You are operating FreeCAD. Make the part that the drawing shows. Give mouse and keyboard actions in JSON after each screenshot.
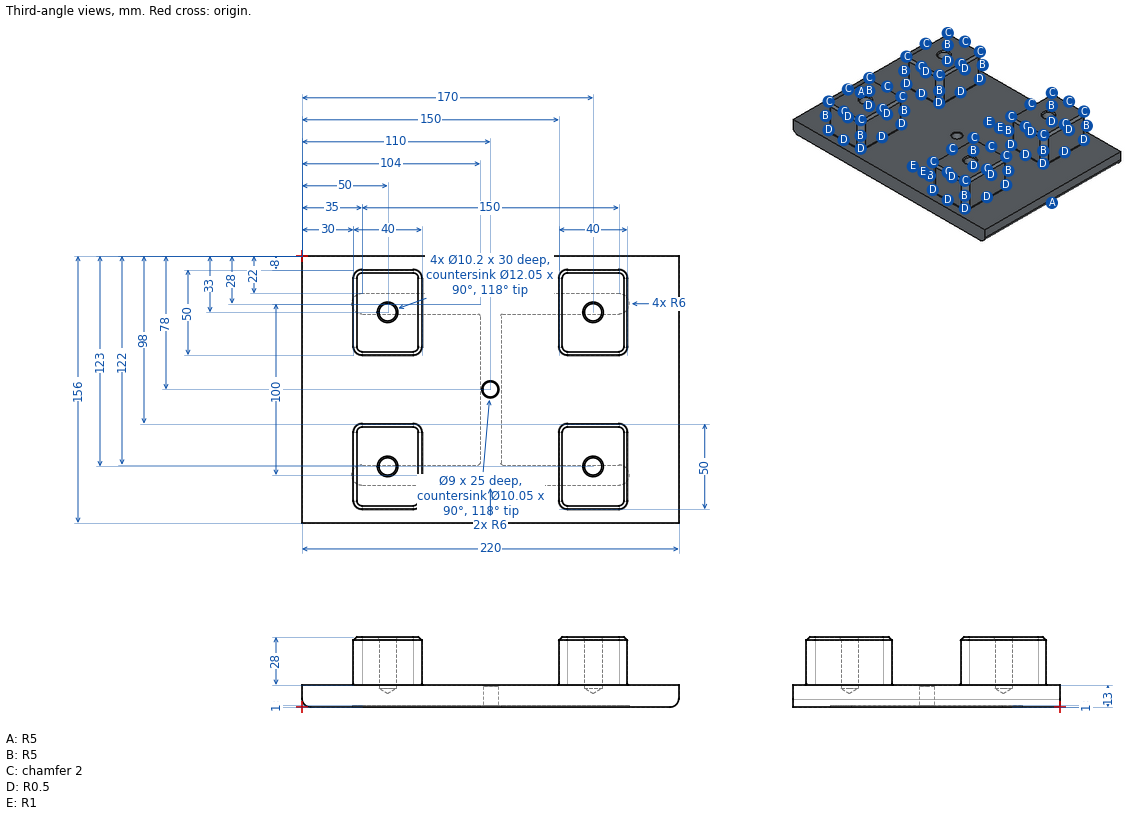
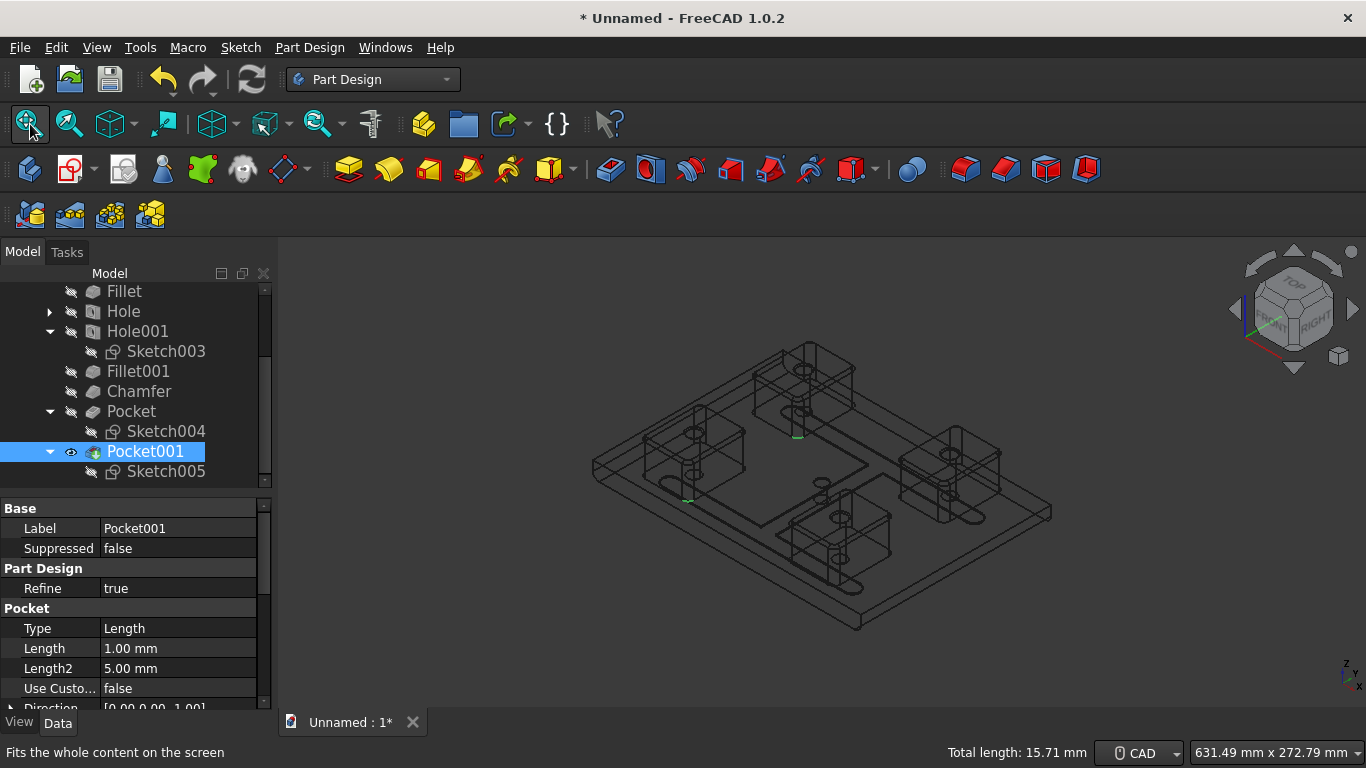
{"action": "left_click", "coordinate": [725, 453], "text": "ctrl"}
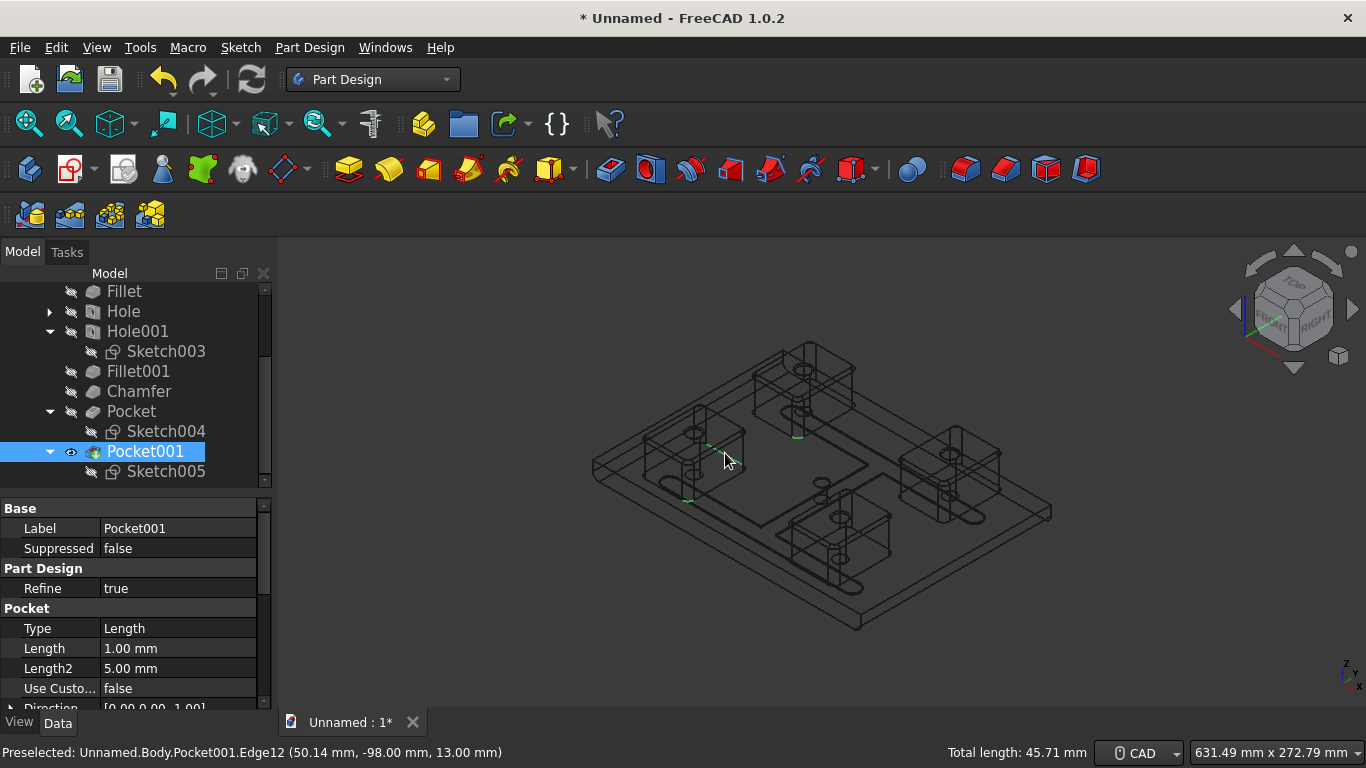
{"action": "left_click", "coordinate": [718, 485], "text": "ctrl"}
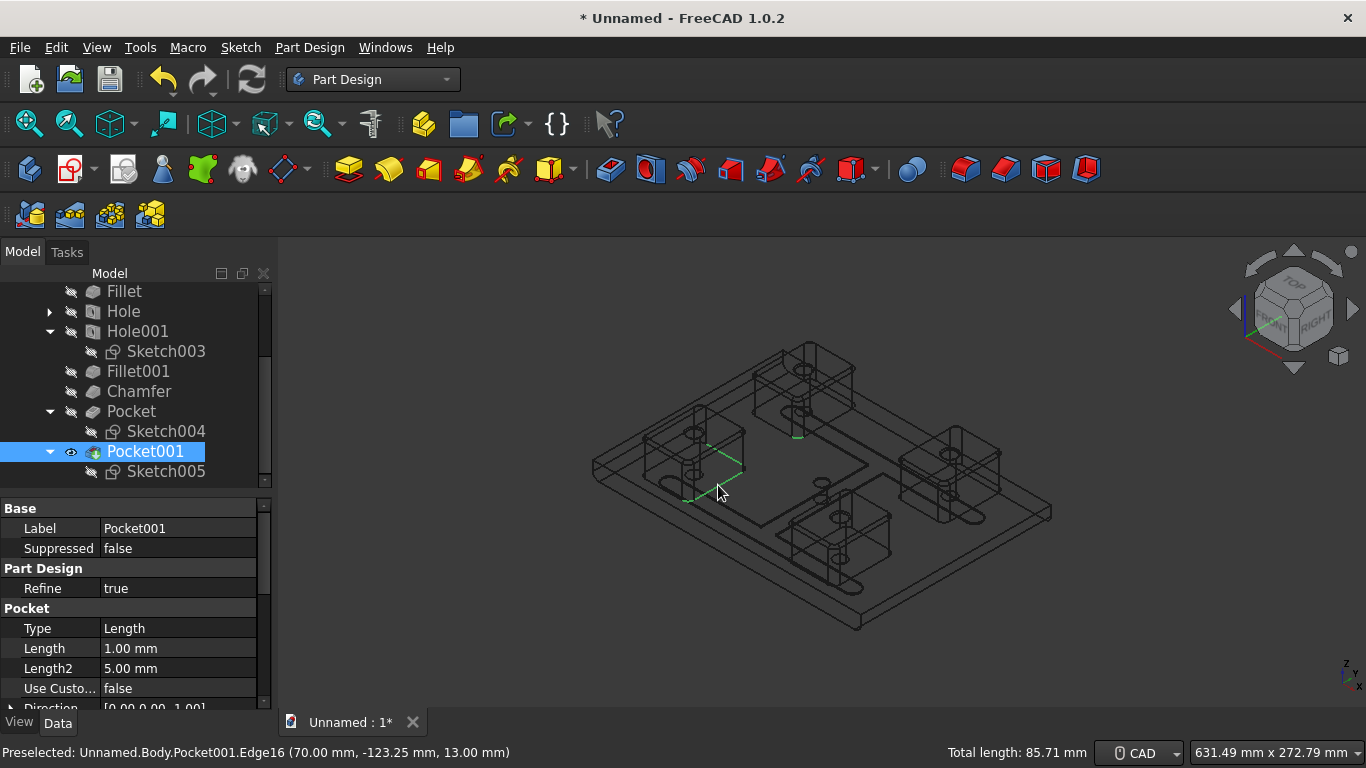
{"action": "left_click", "coordinate": [660, 463], "text": "ctrl"}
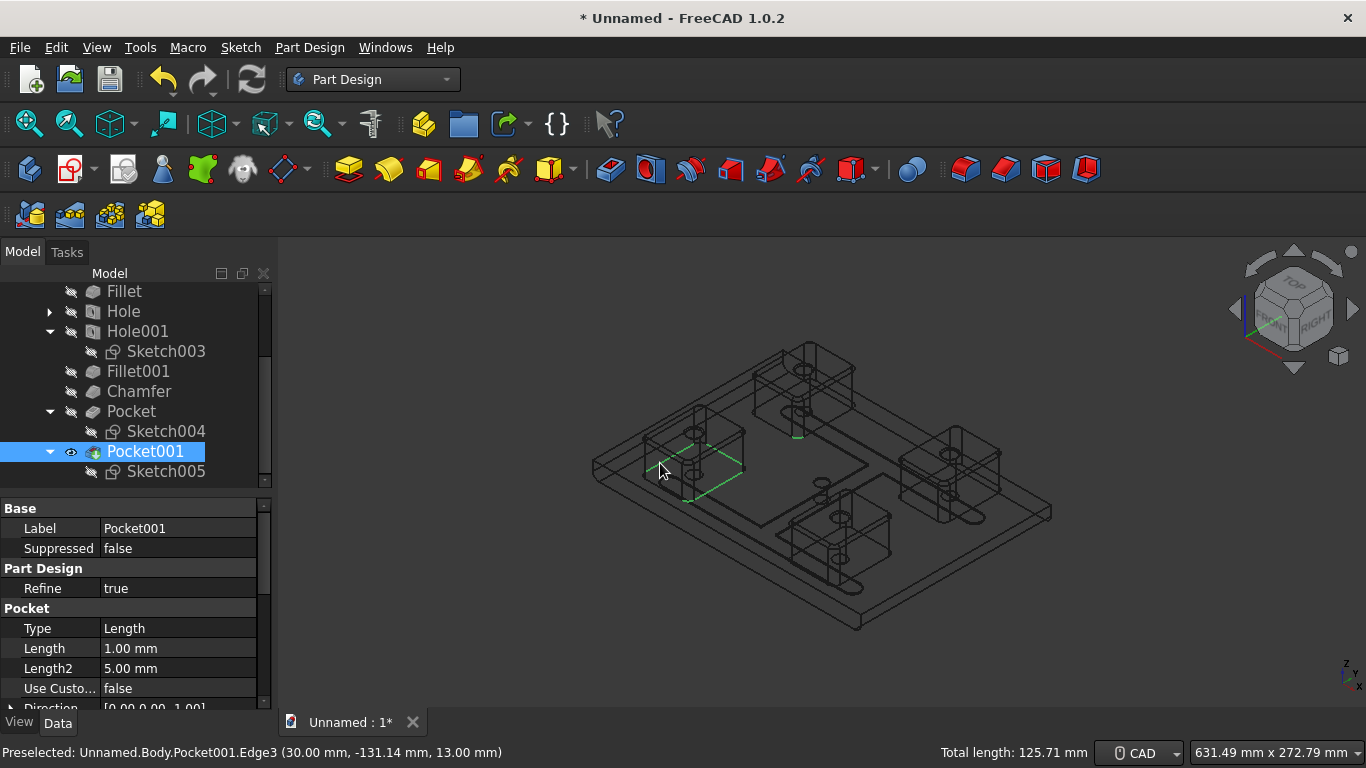
{"action": "left_click", "coordinate": [664, 489], "text": "ctrl"}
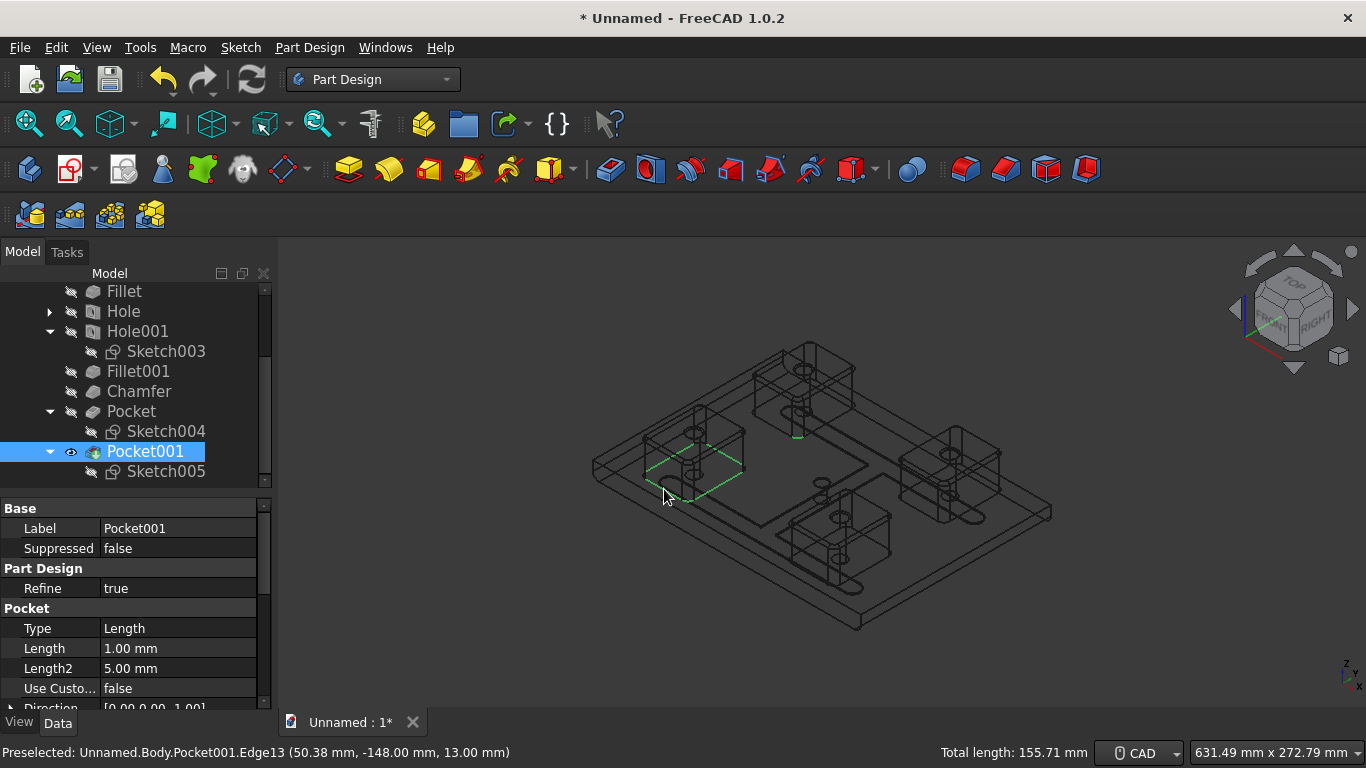
{"action": "left_click", "coordinate": [810, 573], "text": "ctrl"}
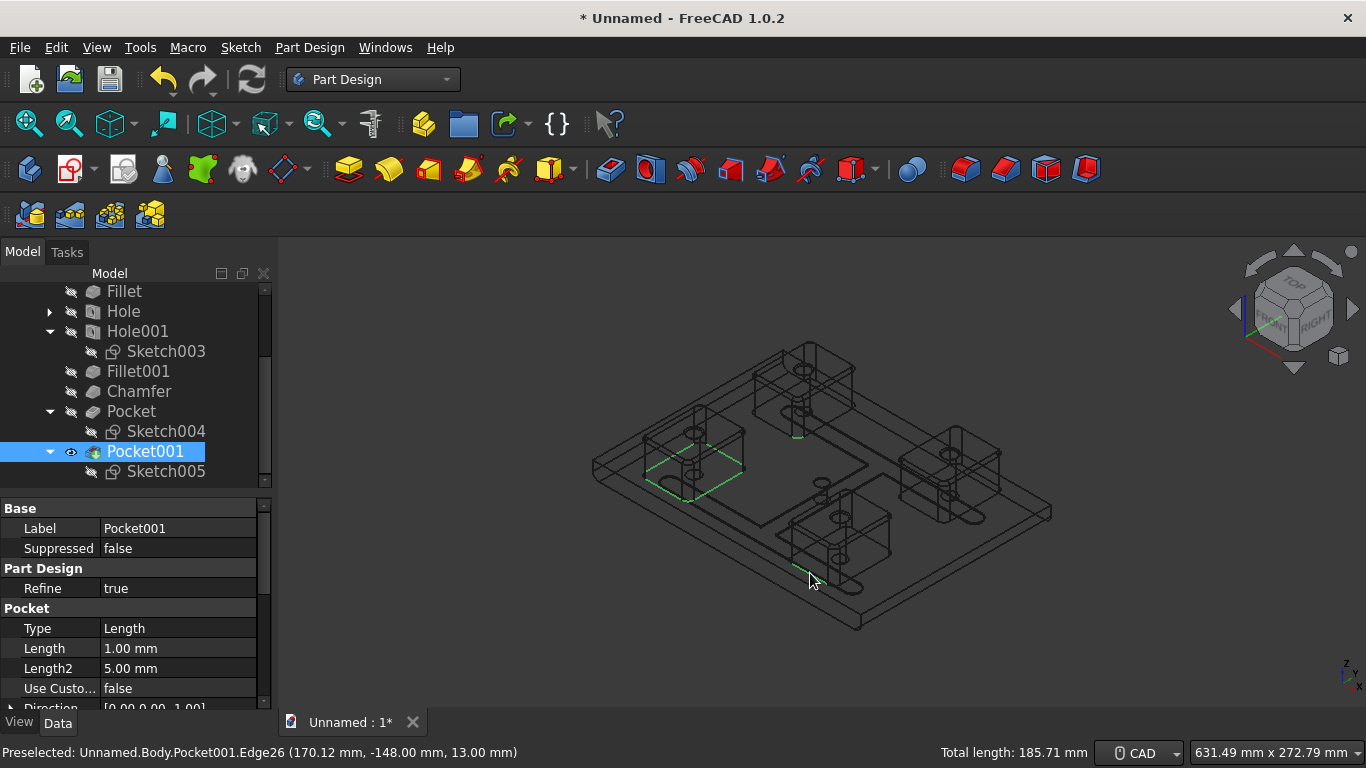
{"action": "left_click", "coordinate": [806, 547], "text": "ctrl"}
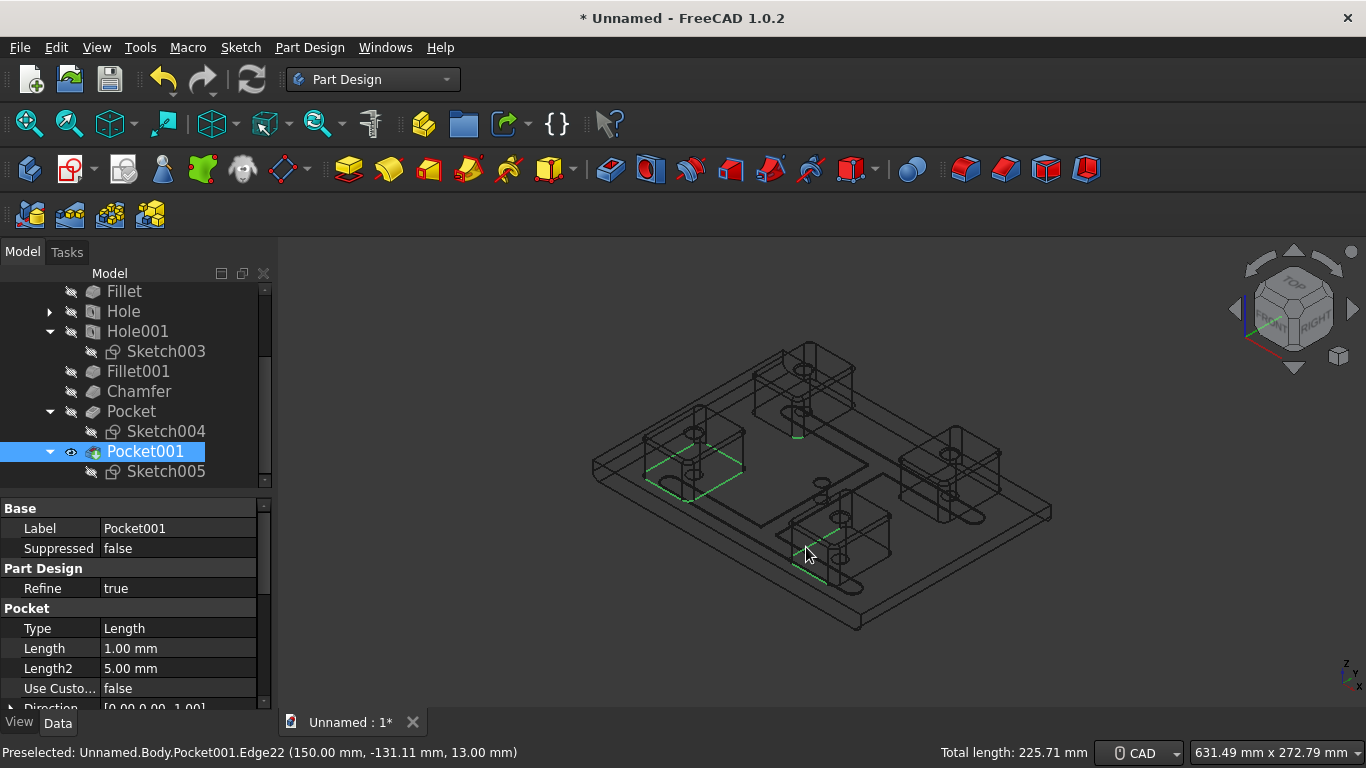
{"action": "left_click", "coordinate": [865, 569], "text": "ctrl"}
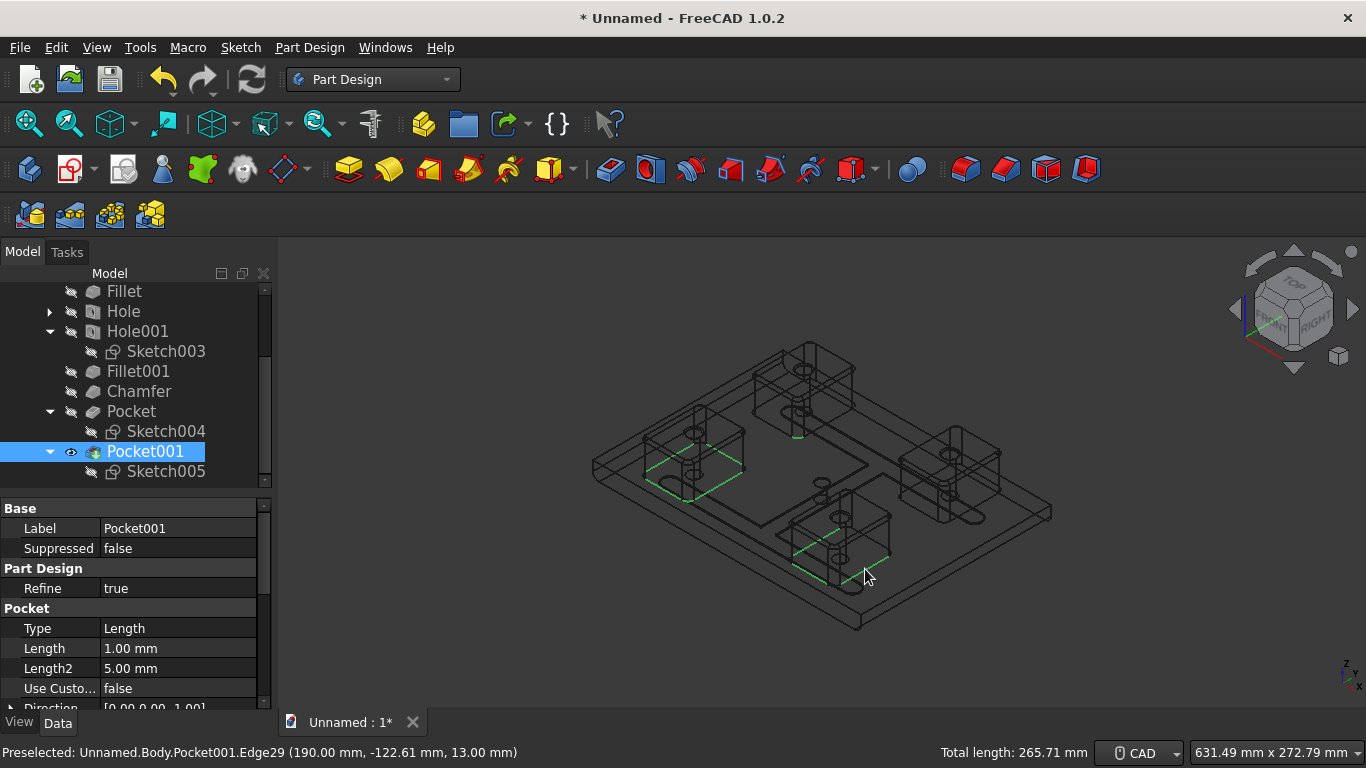
{"action": "left_click", "coordinate": [871, 538], "text": "ctrl"}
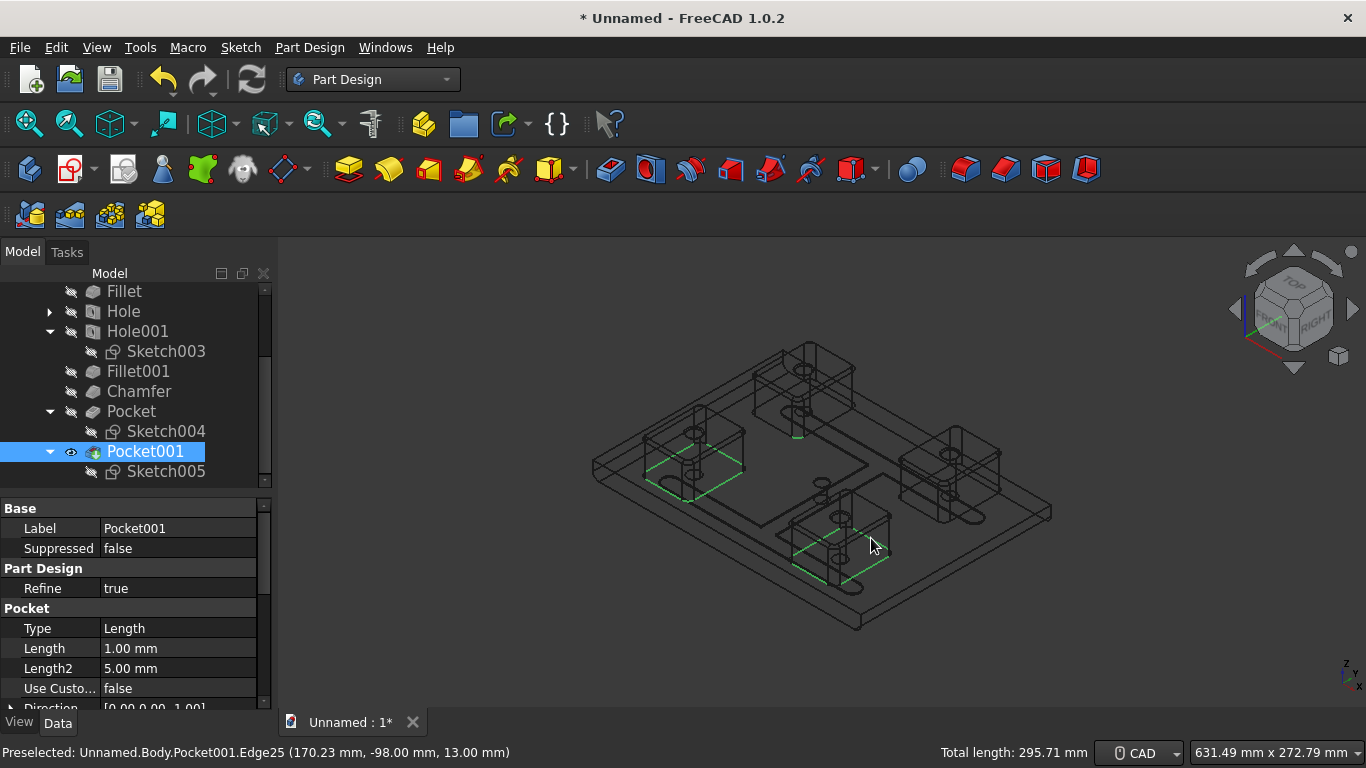
{"action": "left_click", "coordinate": [916, 484], "text": "ctrl"}